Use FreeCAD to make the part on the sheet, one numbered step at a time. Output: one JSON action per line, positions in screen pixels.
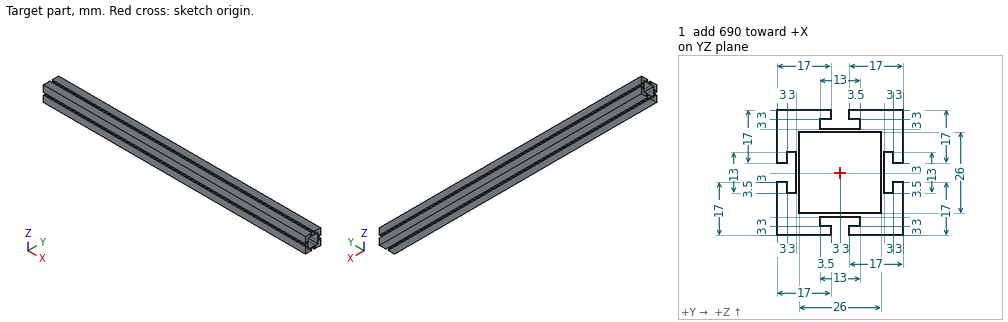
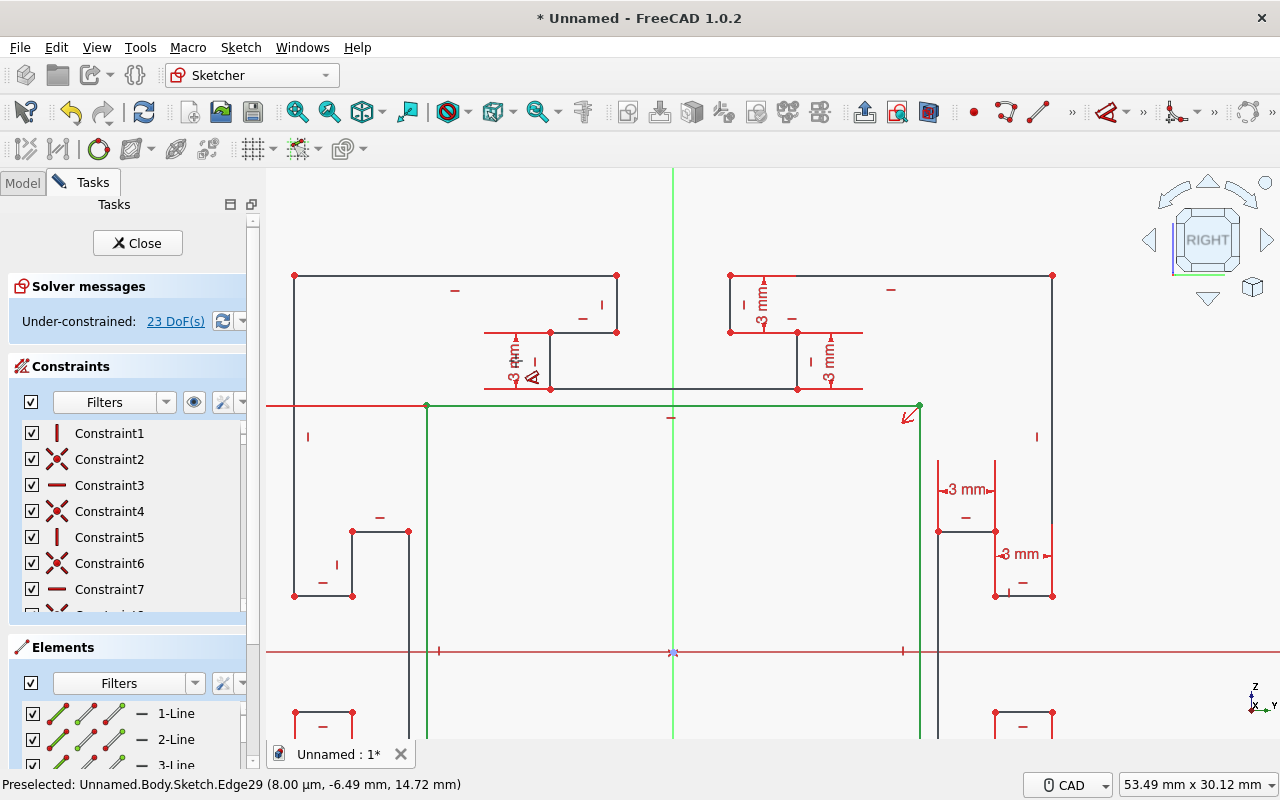
{"action": "left_click", "coordinate": [617, 316]}
{"action": "left_click", "coordinate": [583, 304]}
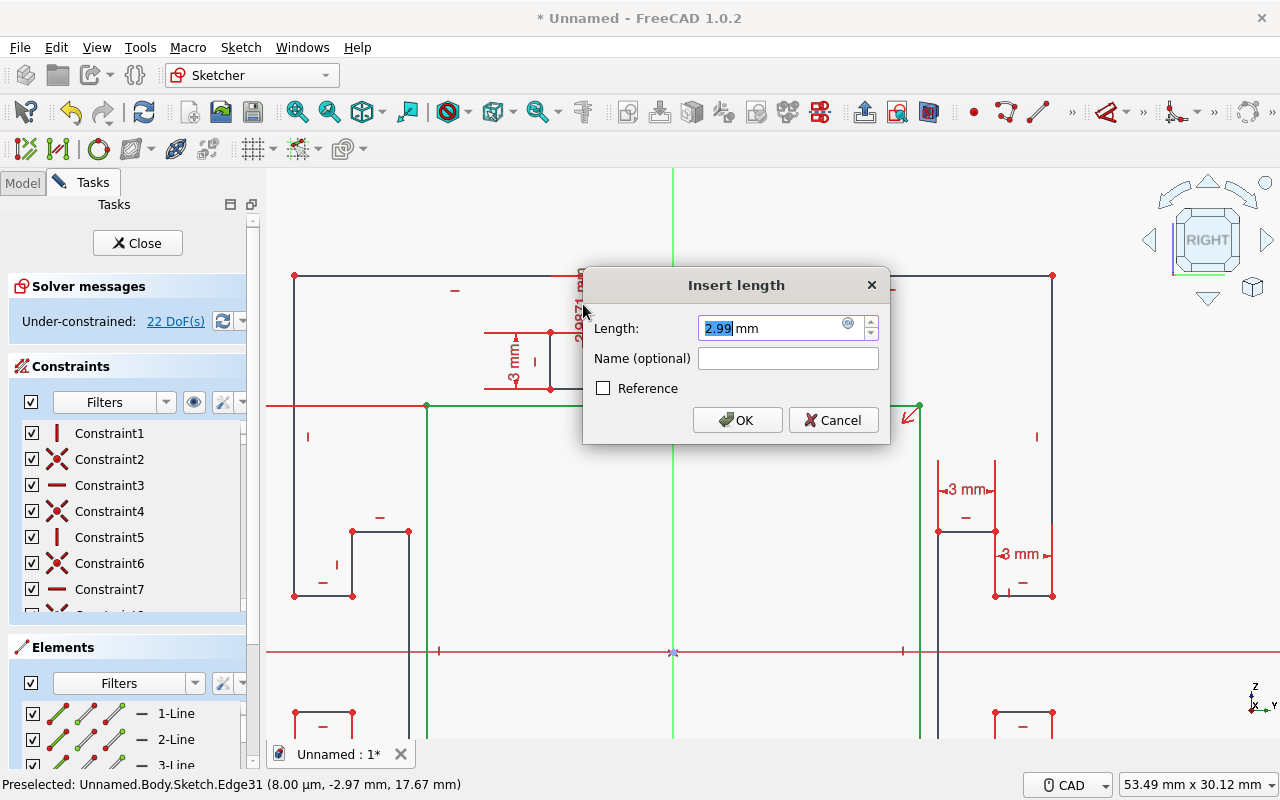
{"action": "type", "text": "3"}
{"action": "key", "text": "Return"}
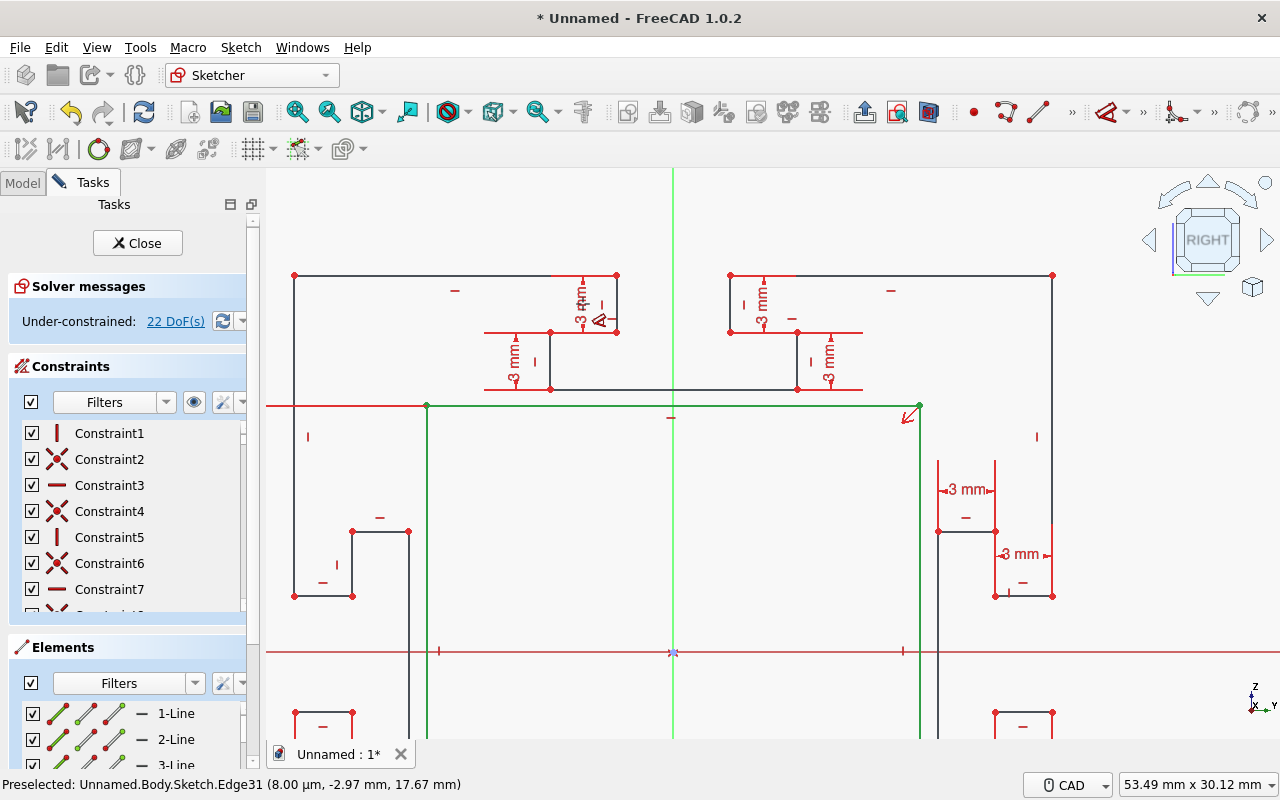
{"action": "left_click", "coordinate": [312, 596]}
{"action": "left_click", "coordinate": [323, 562]}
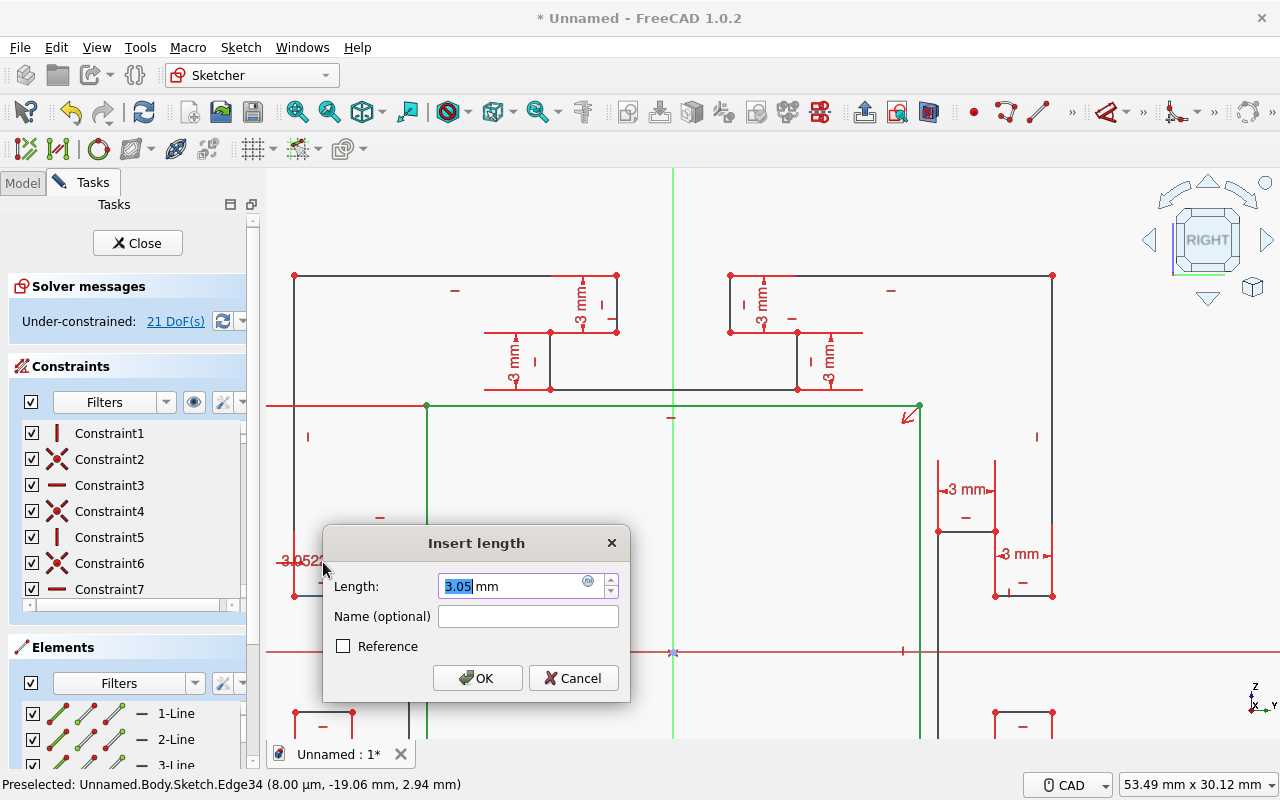
{"action": "type", "text": "3"}
{"action": "key", "text": "Return"}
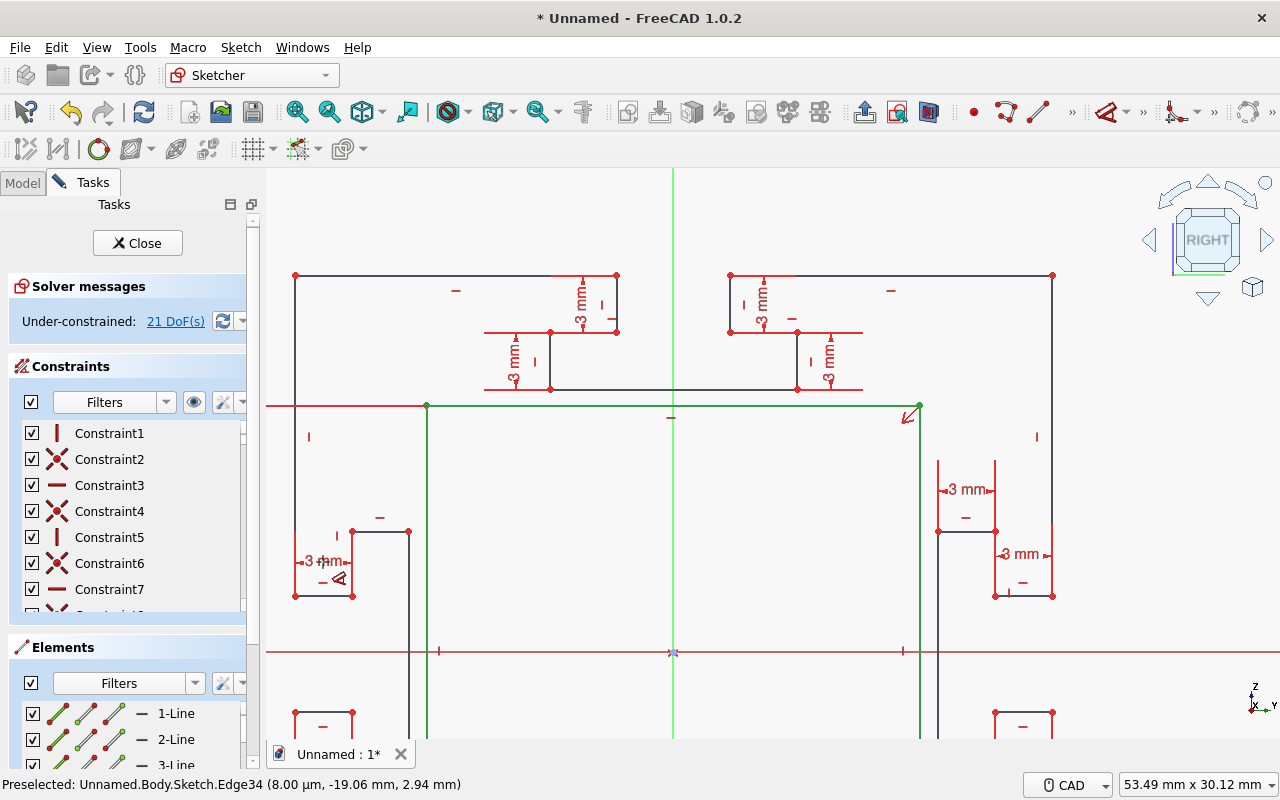
{"action": "left_click", "coordinate": [369, 532]}
{"action": "left_click", "coordinate": [381, 498]}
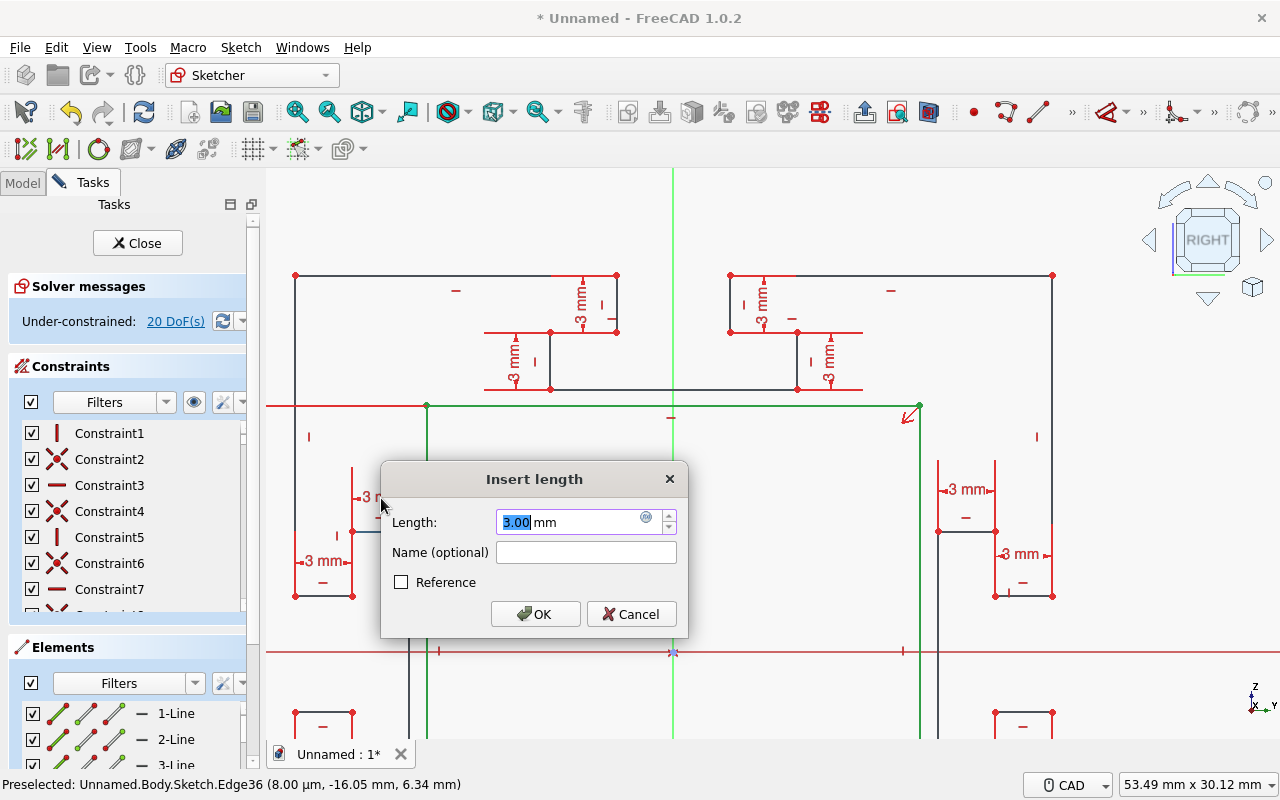
{"action": "type", "text": "3"}
{"action": "key", "text": "Return"}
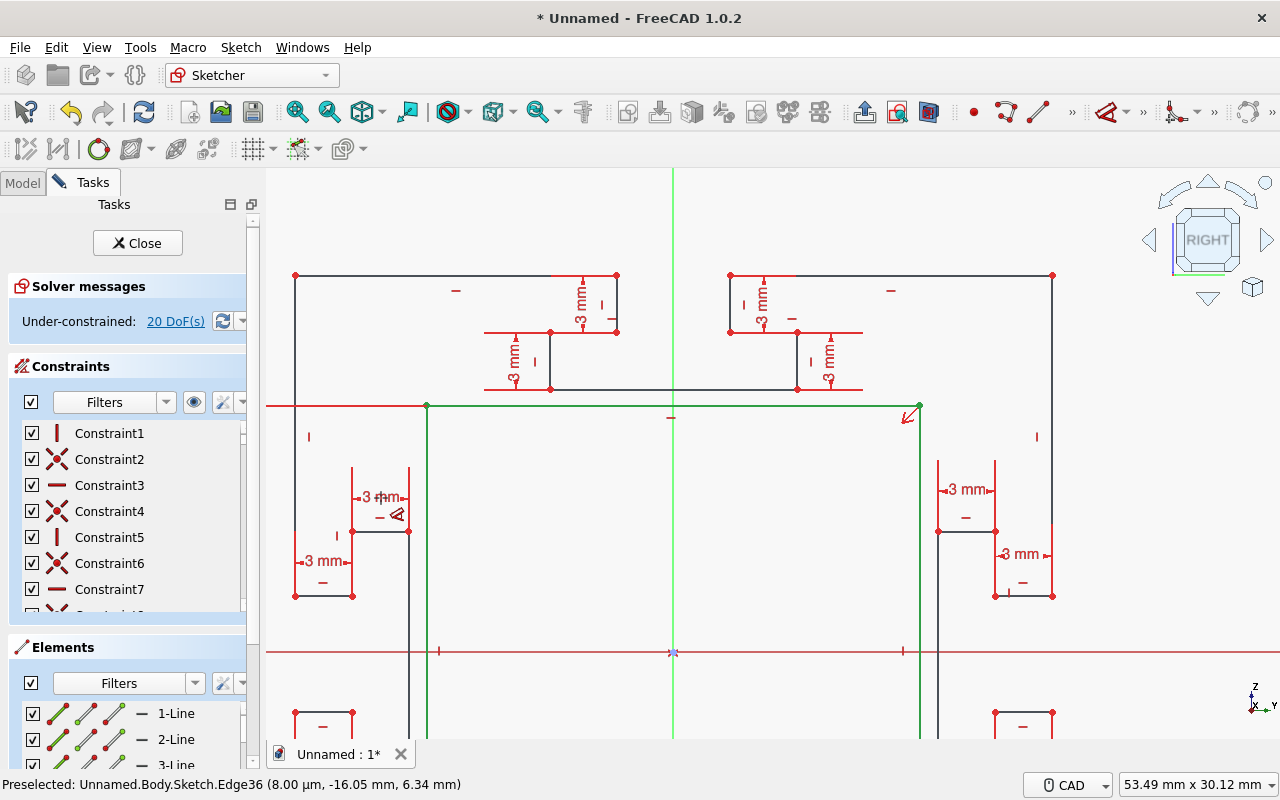
{"action": "left_click", "coordinate": [409, 605]}
{"action": "left_click", "coordinate": [375, 621]}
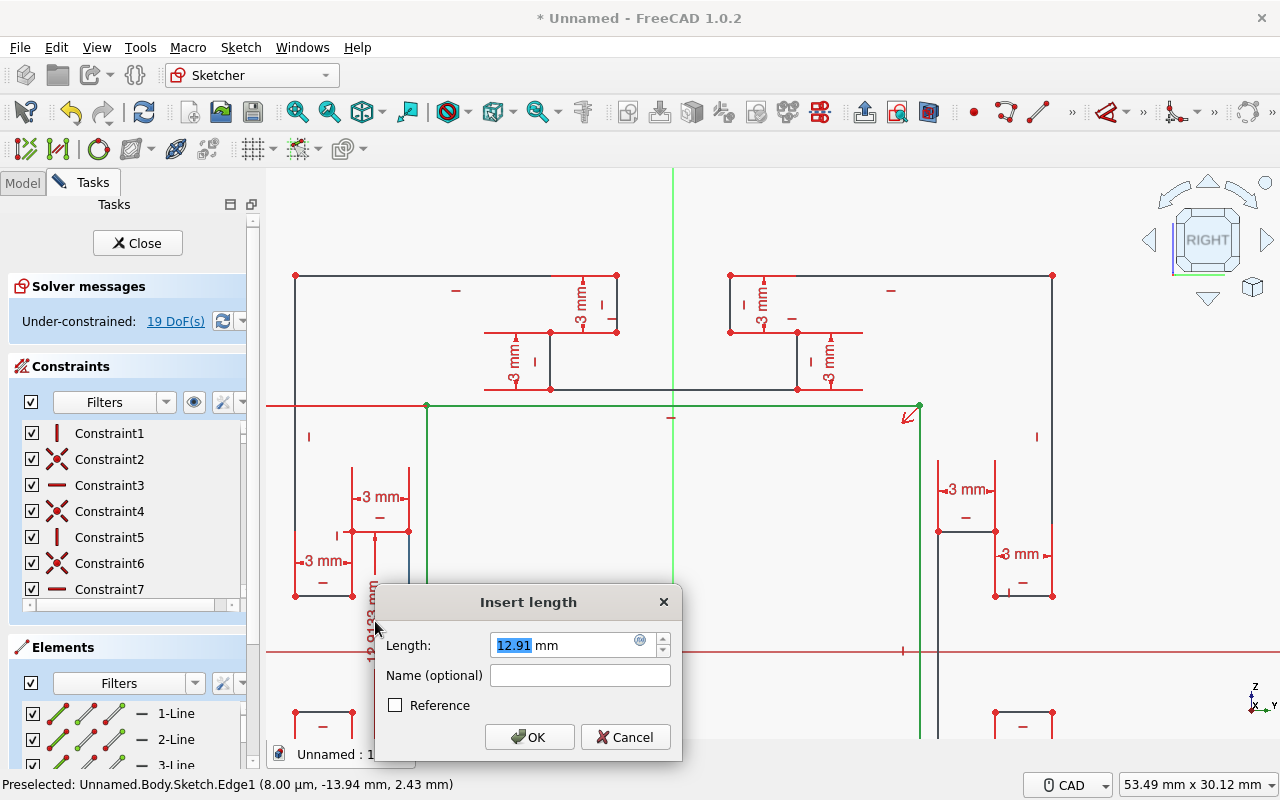
{"action": "type", "text": "13"}
{"action": "key", "text": "Return"}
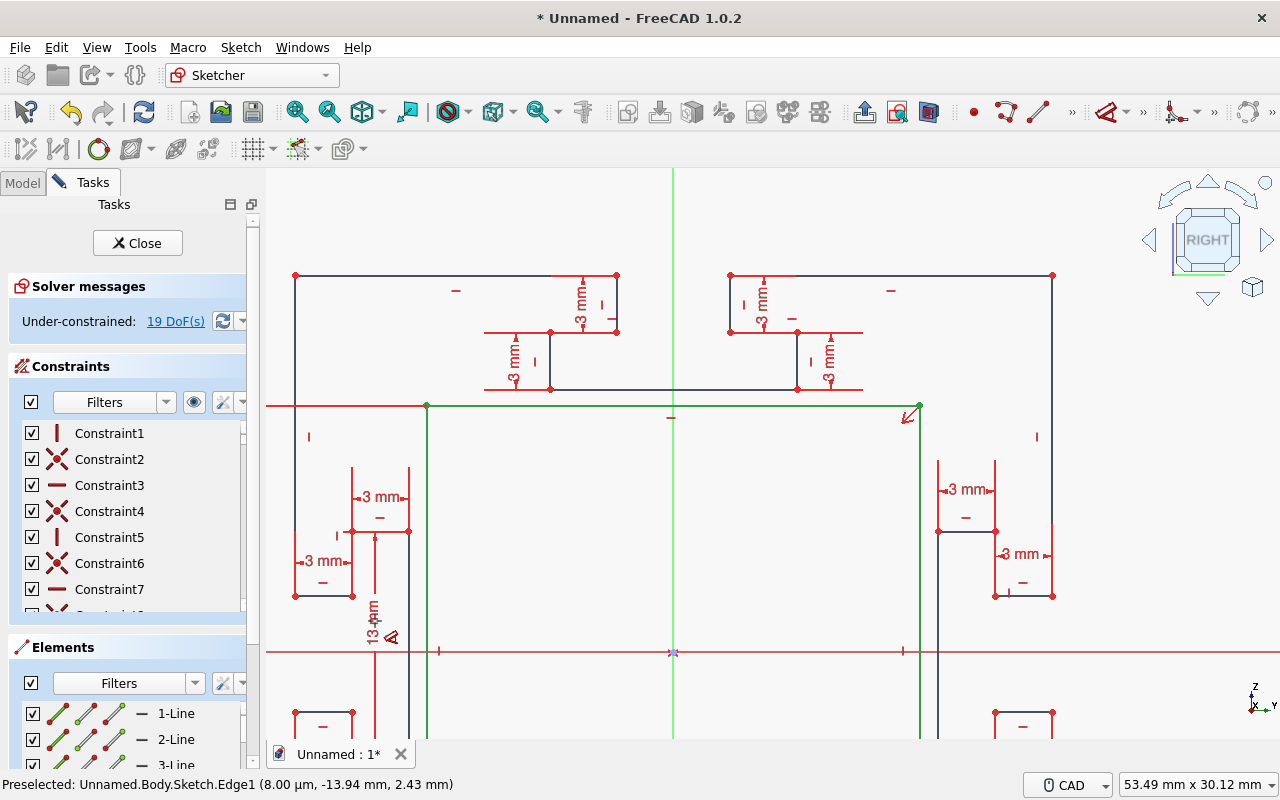
{"action": "scroll", "coordinate": [730, 291], "scroll_direction": "down", "scroll_amount": 4}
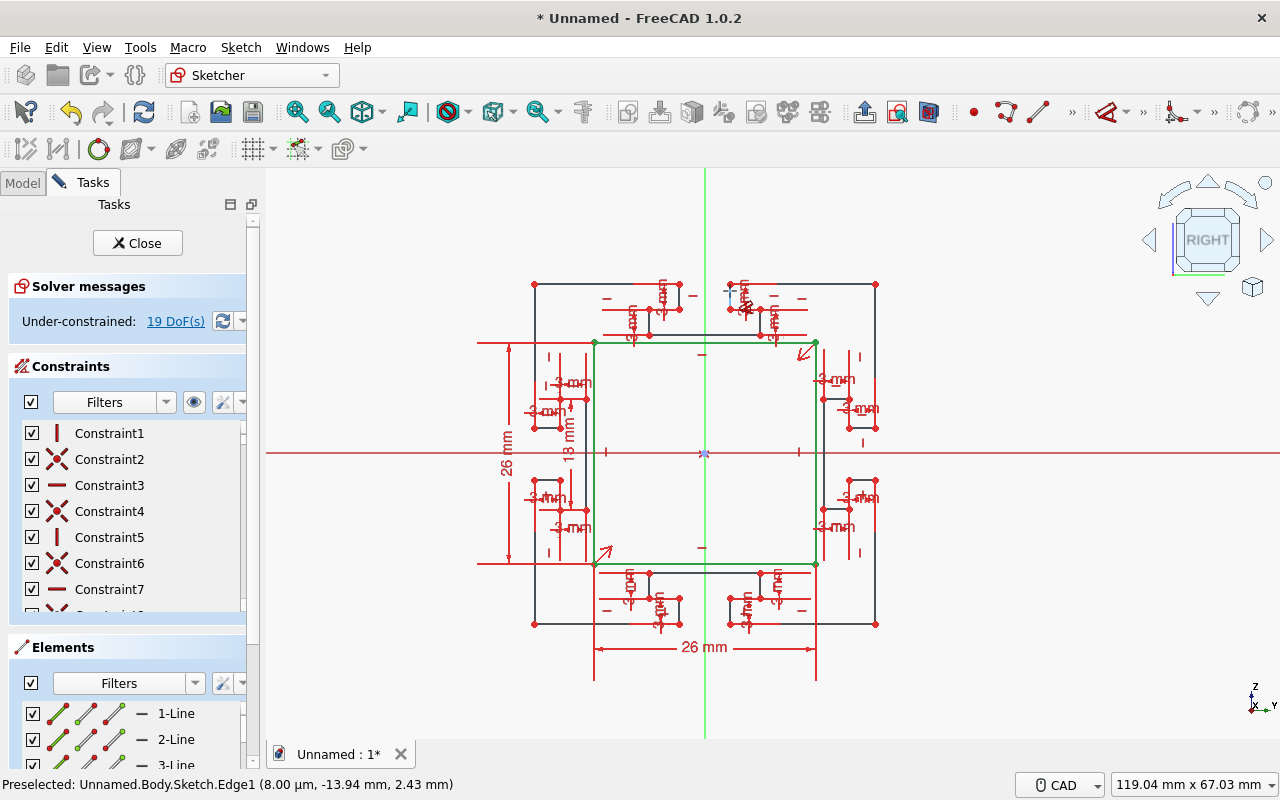
{"action": "left_click", "coordinate": [535, 524]}
{"action": "left_click", "coordinate": [501, 552]}